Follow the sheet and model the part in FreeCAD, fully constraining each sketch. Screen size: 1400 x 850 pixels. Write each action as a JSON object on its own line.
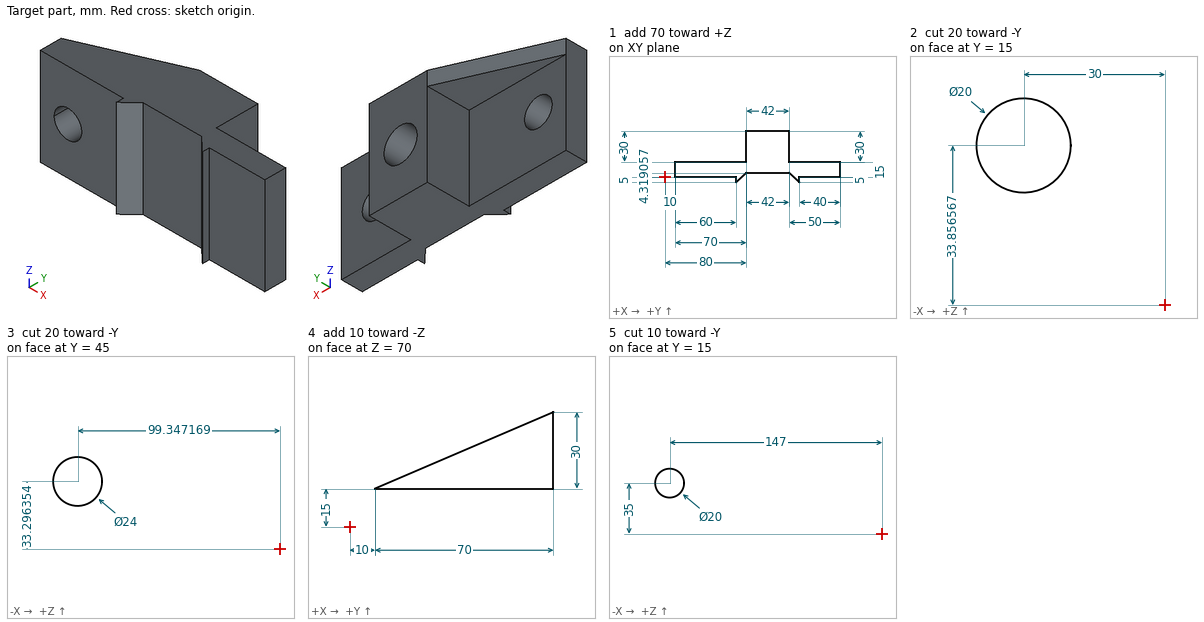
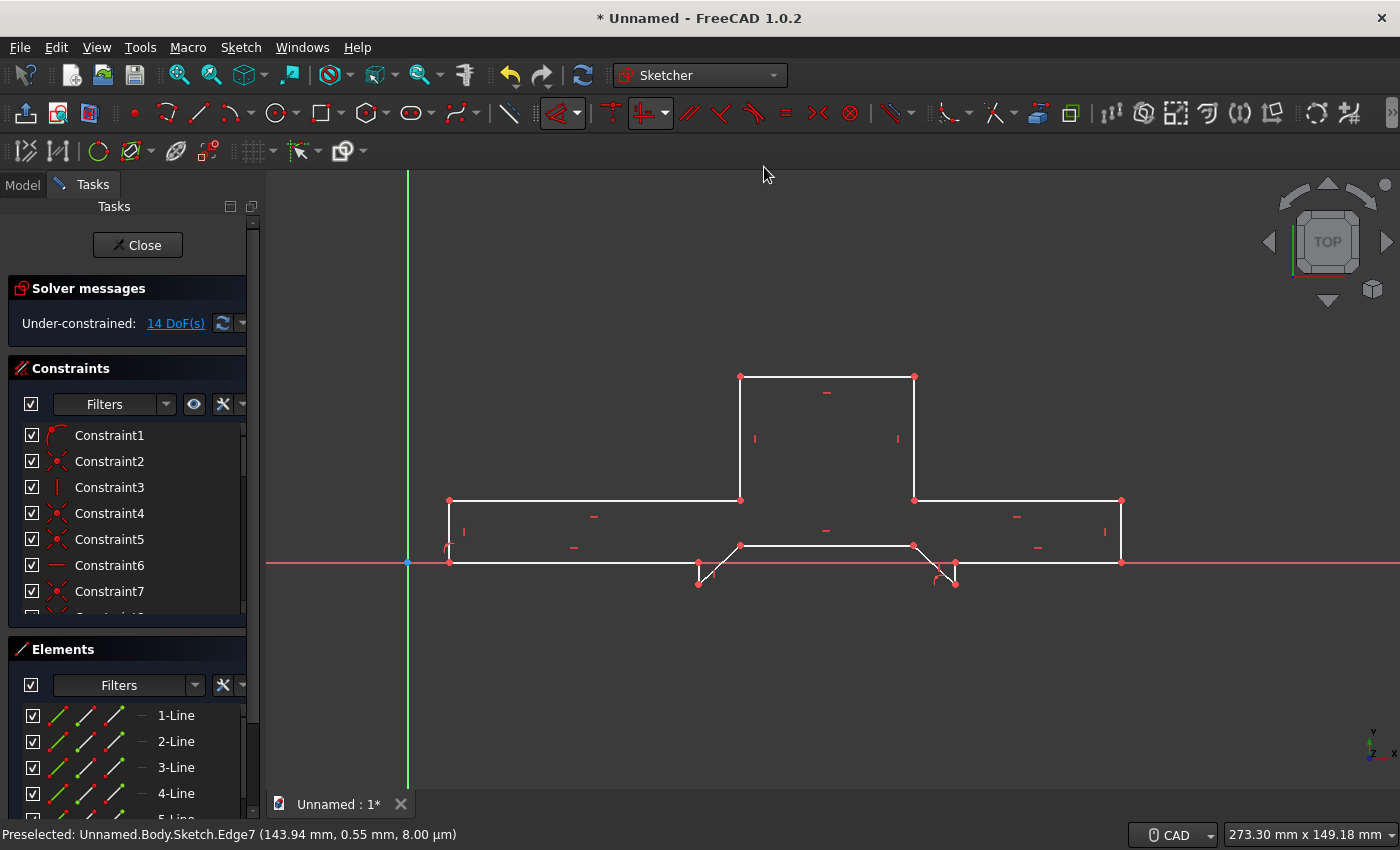
{"action": "left_click", "coordinate": [556, 114]}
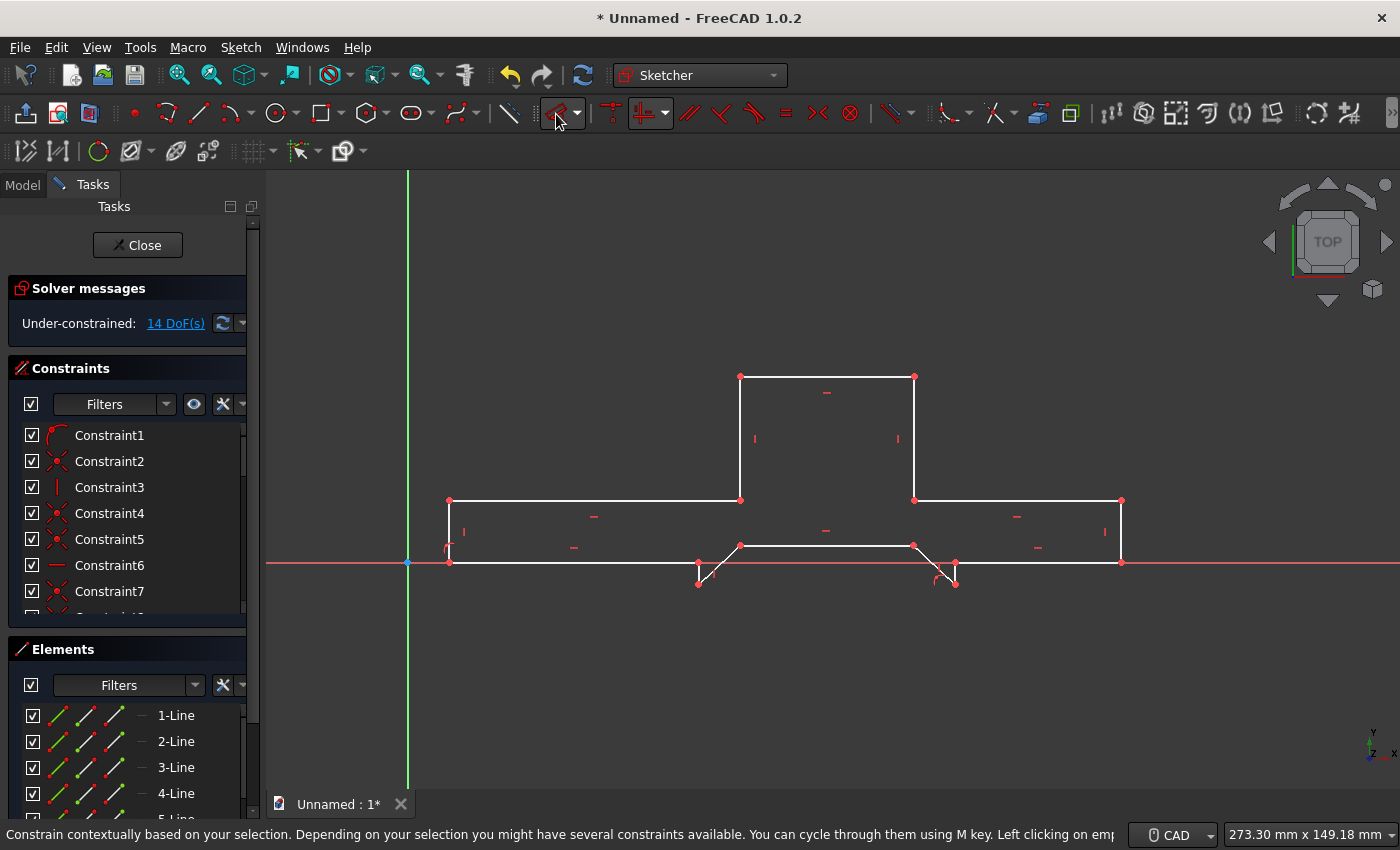
{"action": "scroll", "coordinate": [699, 572], "scroll_direction": "up", "scroll_amount": 4}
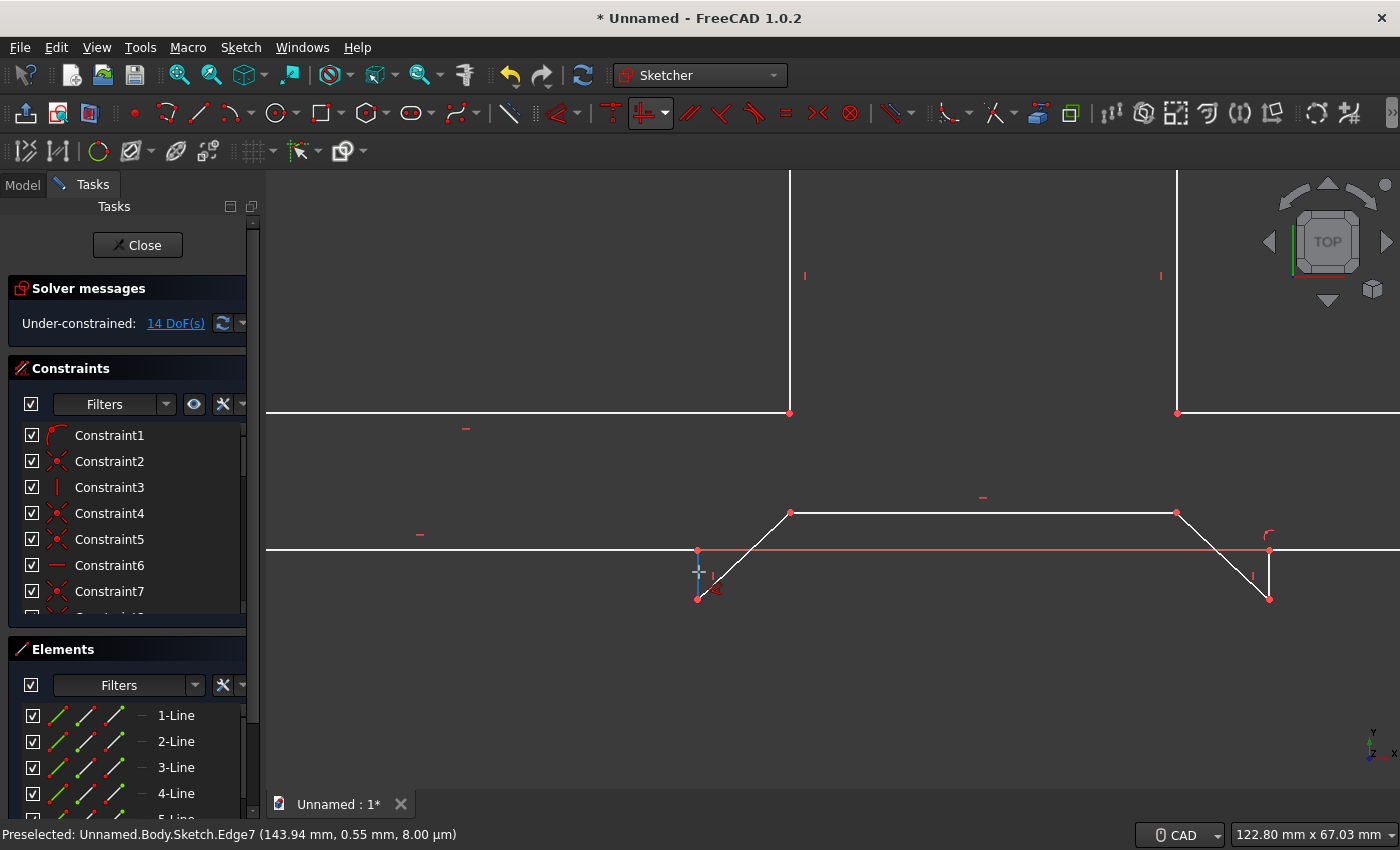
{"action": "left_click", "coordinate": [698, 570]}
{"action": "left_click", "coordinate": [664, 575]}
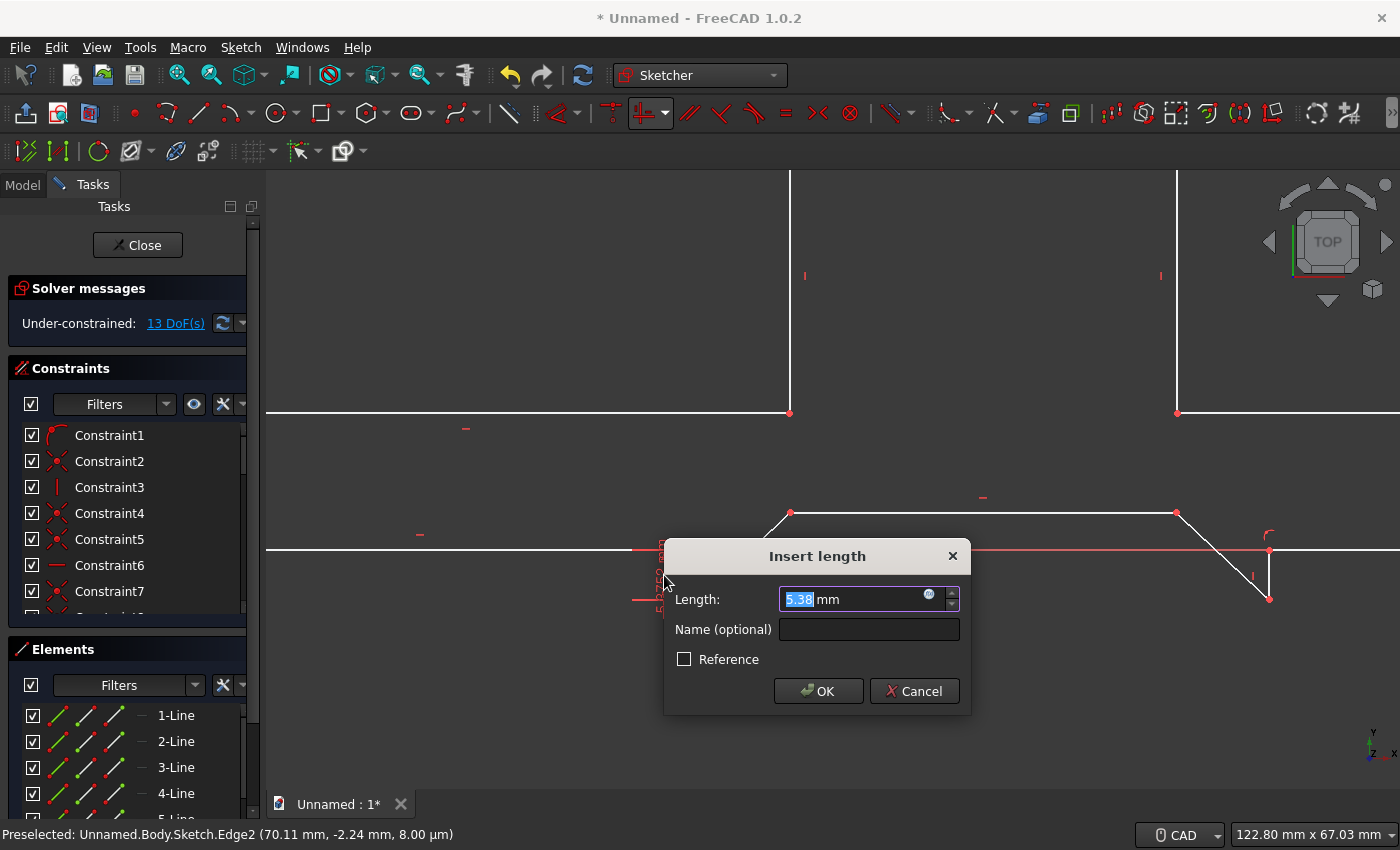
{"action": "type", "text": "5"}
{"action": "key", "text": "Return"}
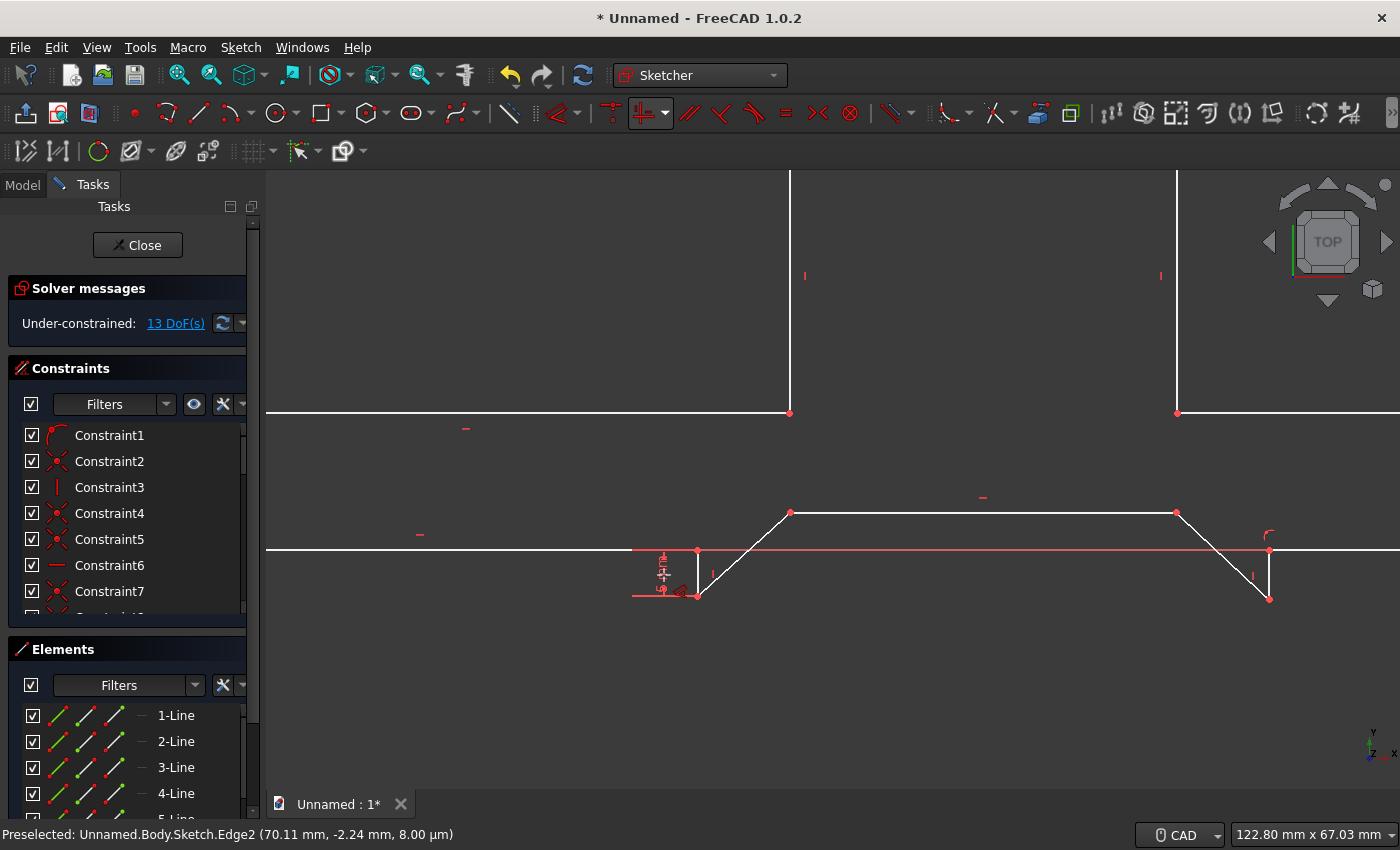
{"action": "scroll", "coordinate": [699, 572], "scroll_direction": "down", "scroll_amount": 4}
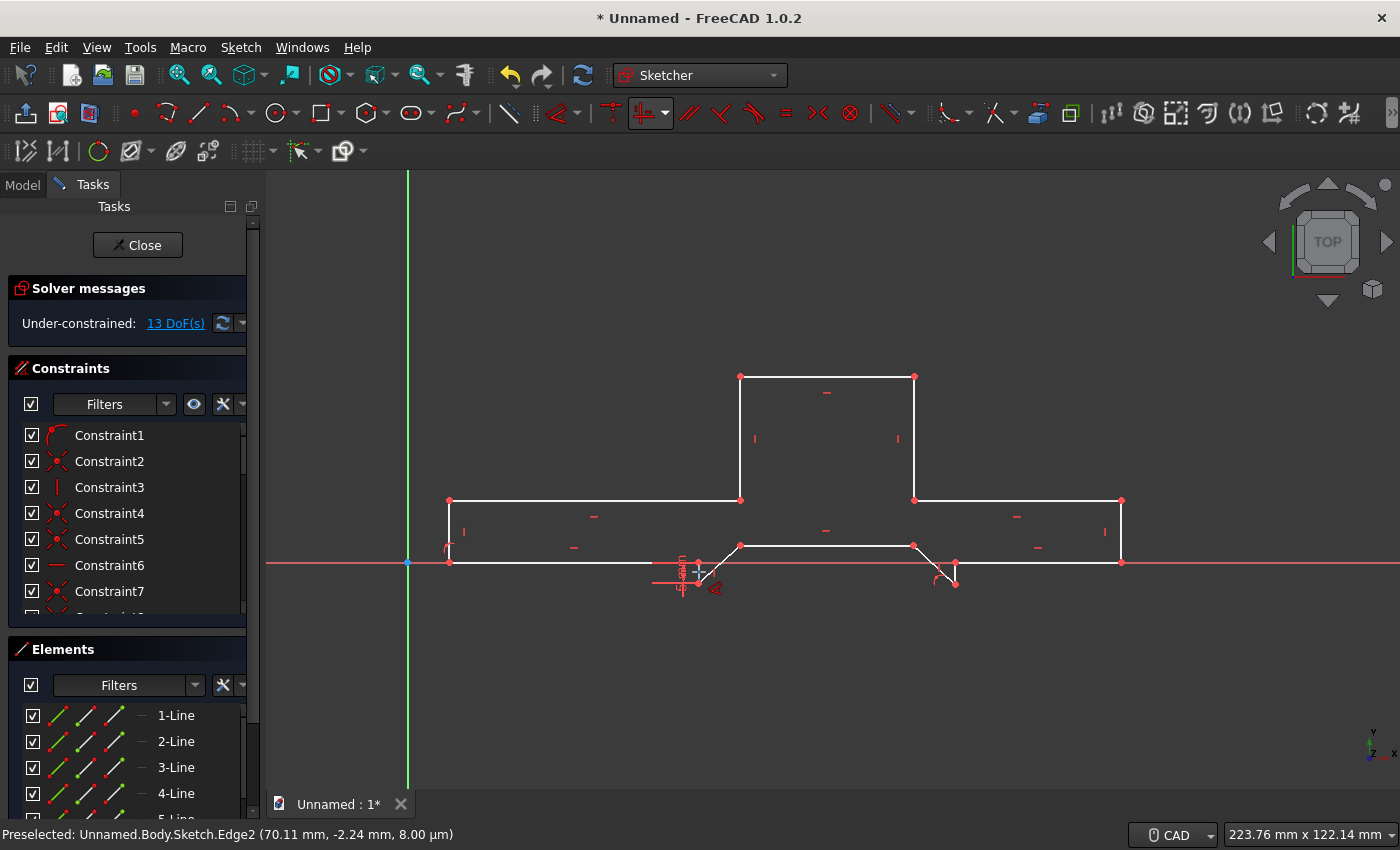
{"action": "scroll", "coordinate": [955, 578], "scroll_direction": "up", "scroll_amount": 6}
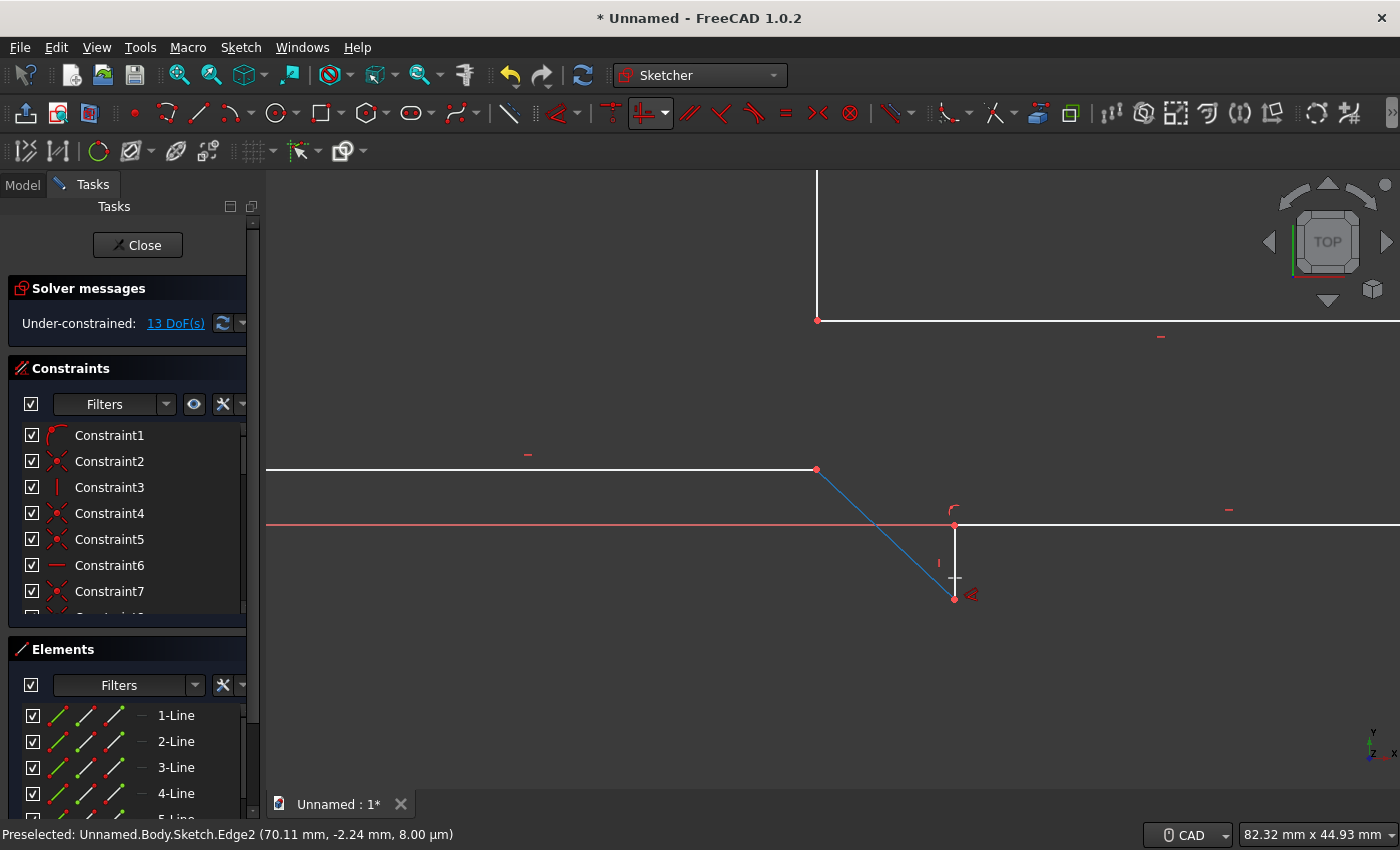
{"action": "left_click", "coordinate": [955, 577]}
{"action": "left_click", "coordinate": [989, 562]}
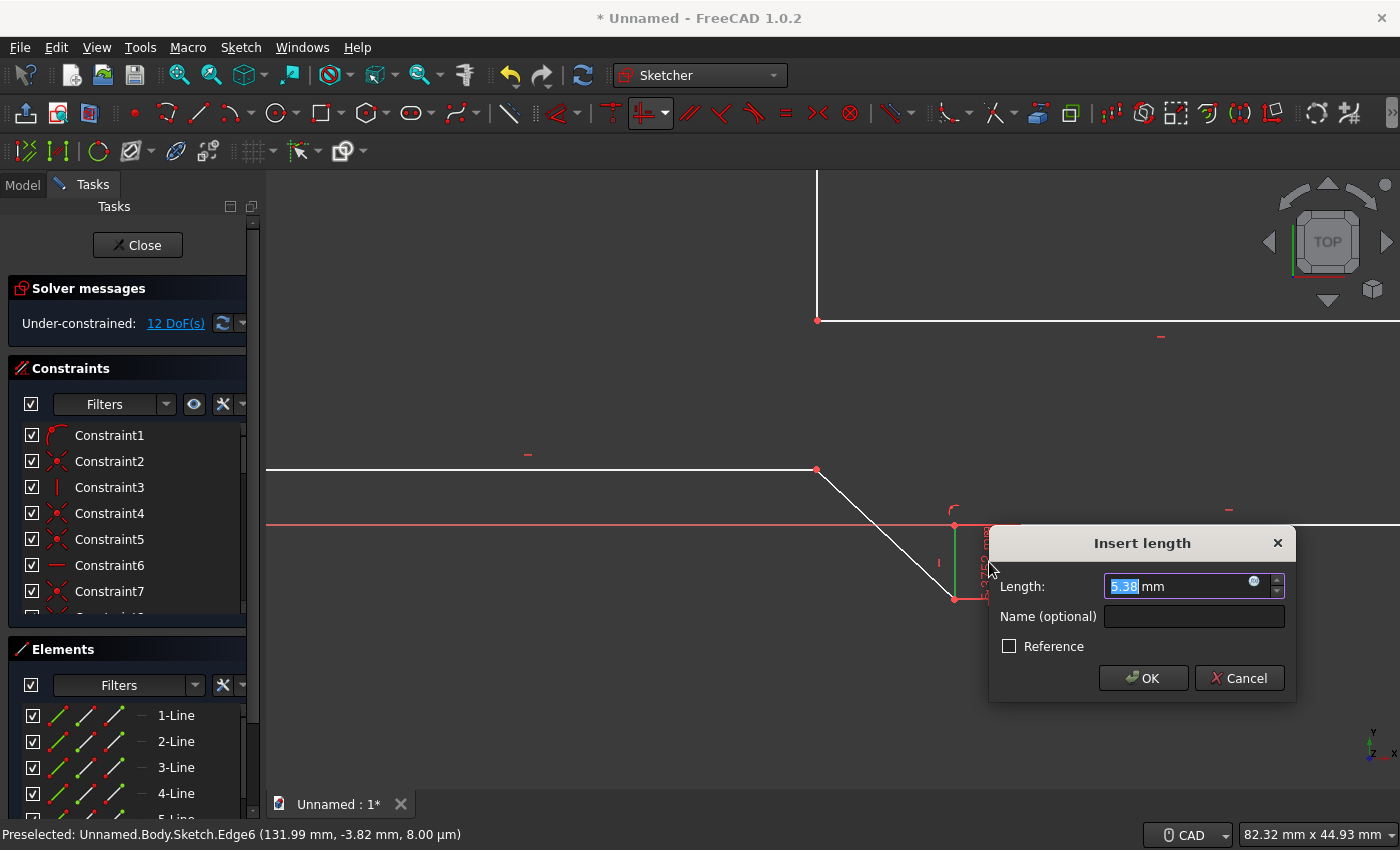
{"action": "type", "text": "5"}
{"action": "key", "text": "Return"}